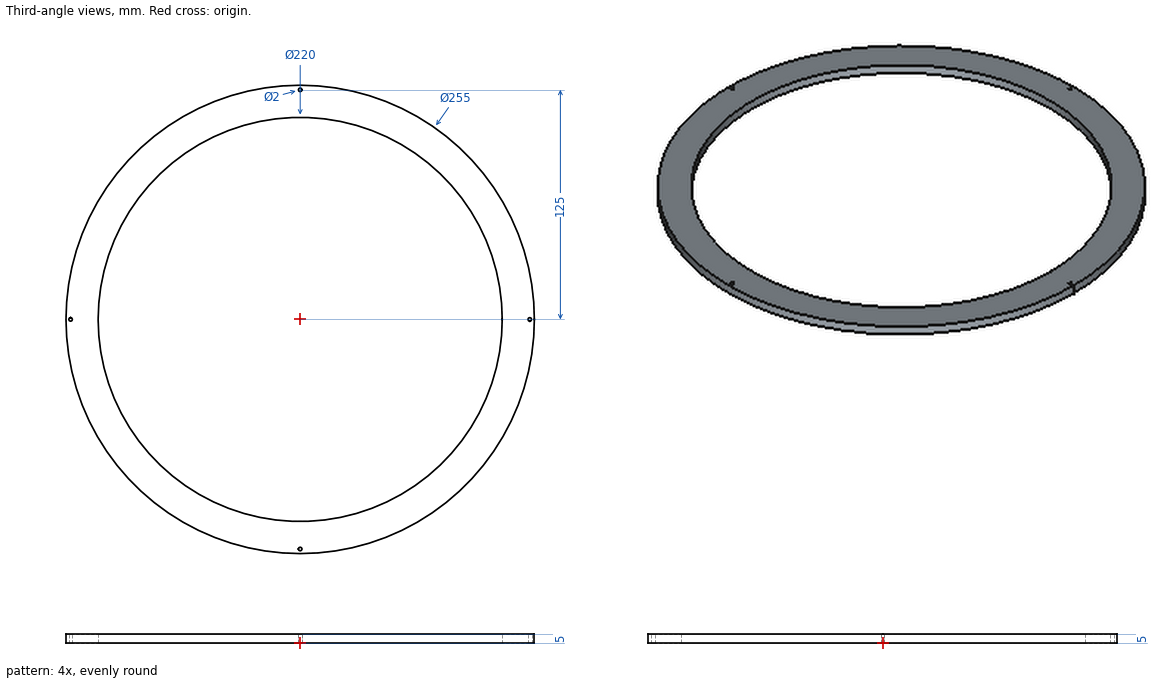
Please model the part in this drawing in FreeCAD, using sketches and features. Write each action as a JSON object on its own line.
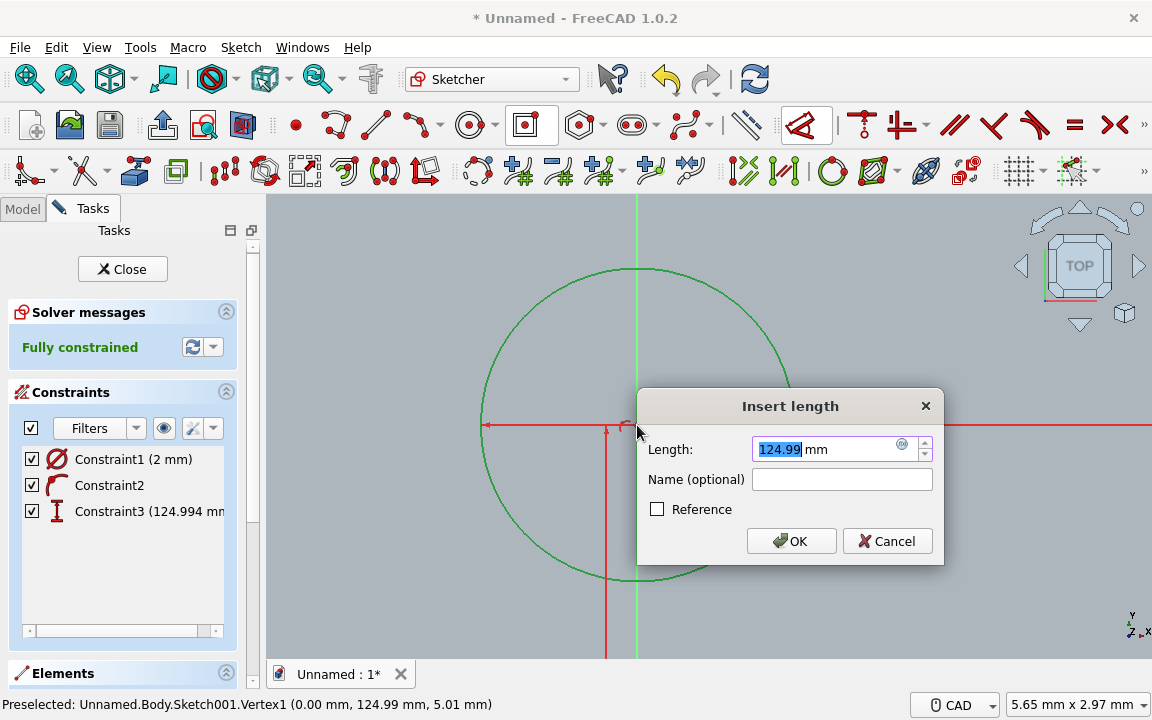
{"action": "type", "text": "125"}
{"action": "key", "text": "Return"}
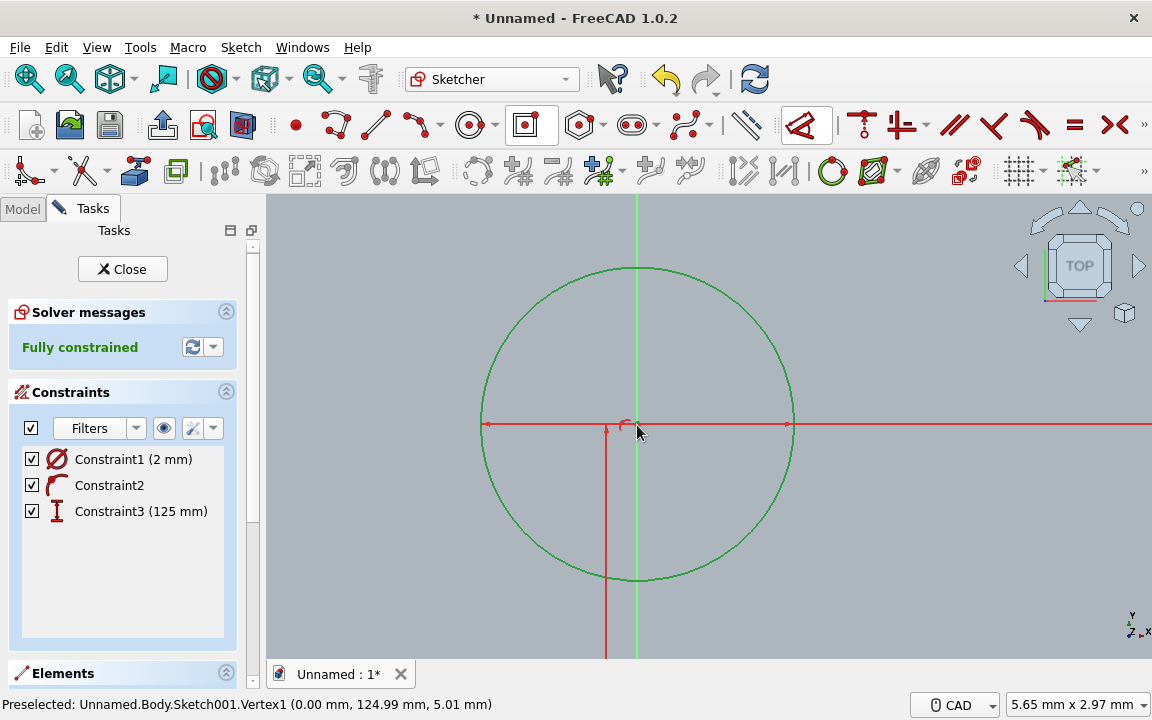
{"action": "left_click", "coordinate": [123, 269]}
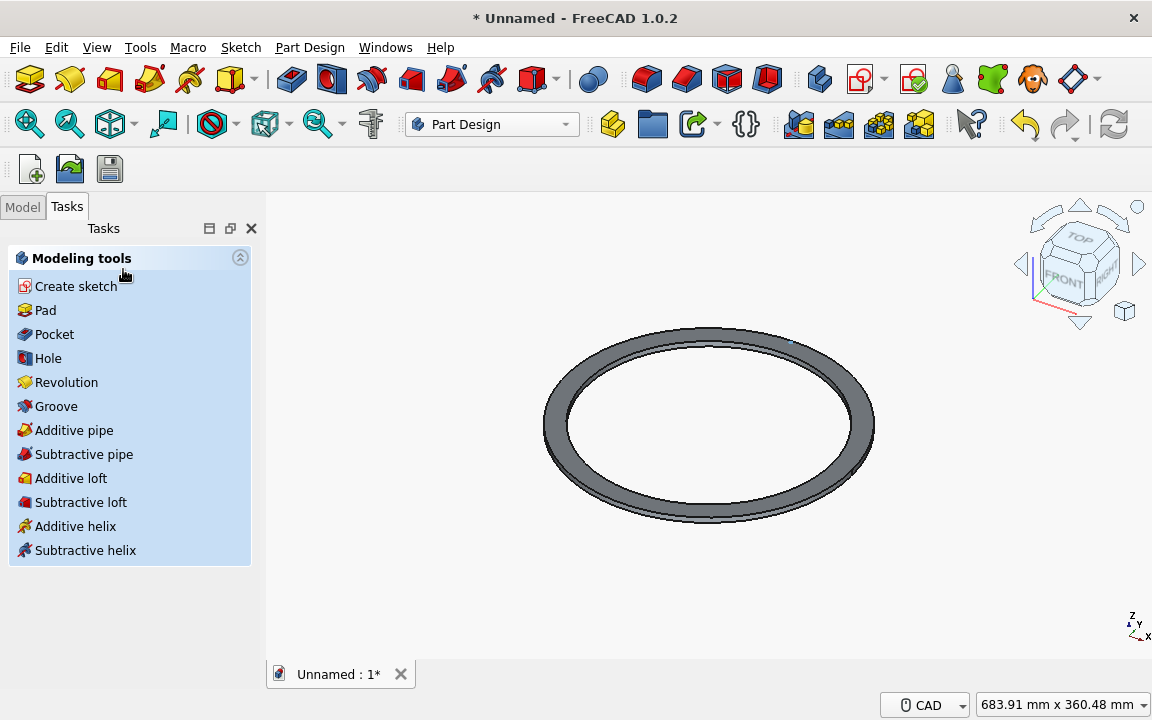
{"action": "left_click", "coordinate": [292, 80]}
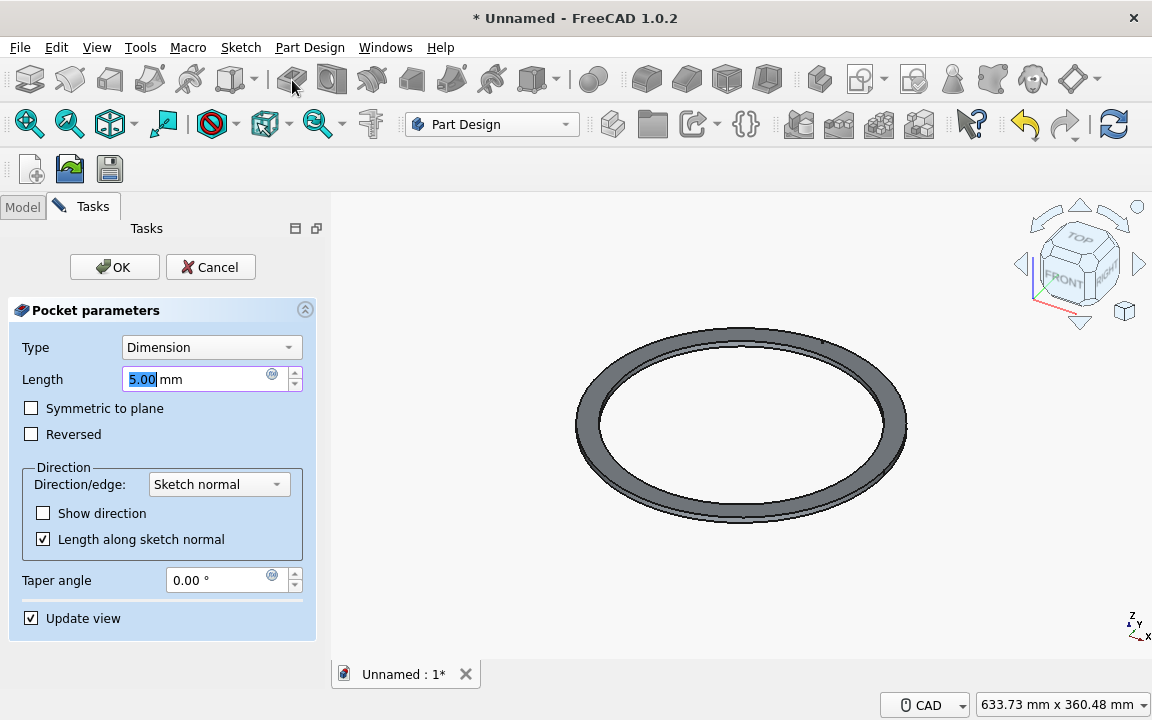
{"action": "type", "text": "5"}
{"action": "key", "text": "Tab"}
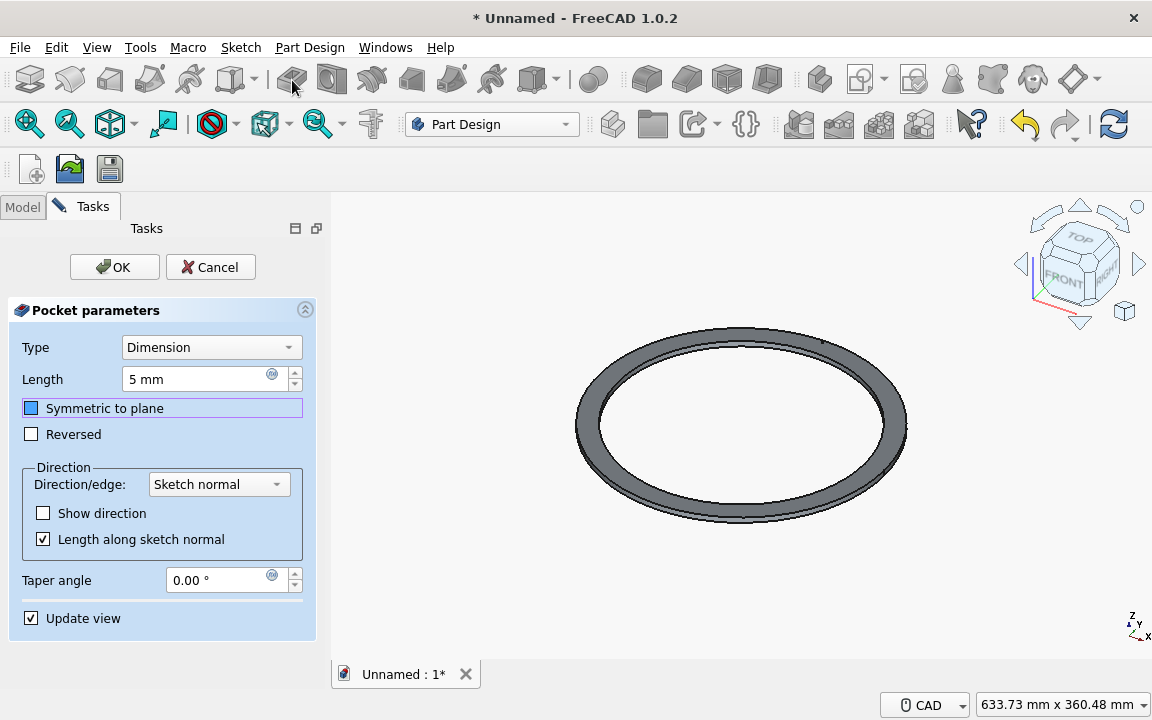
{"action": "left_click", "coordinate": [115, 267]}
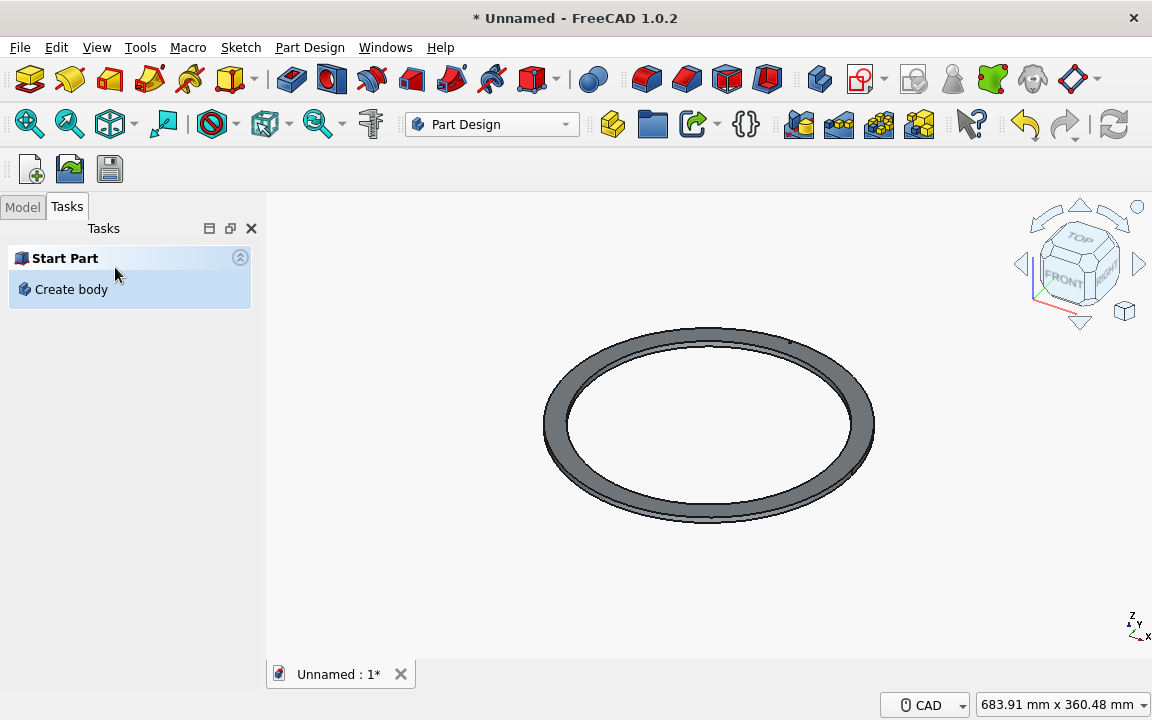
{"action": "left_click", "coordinate": [23, 206]}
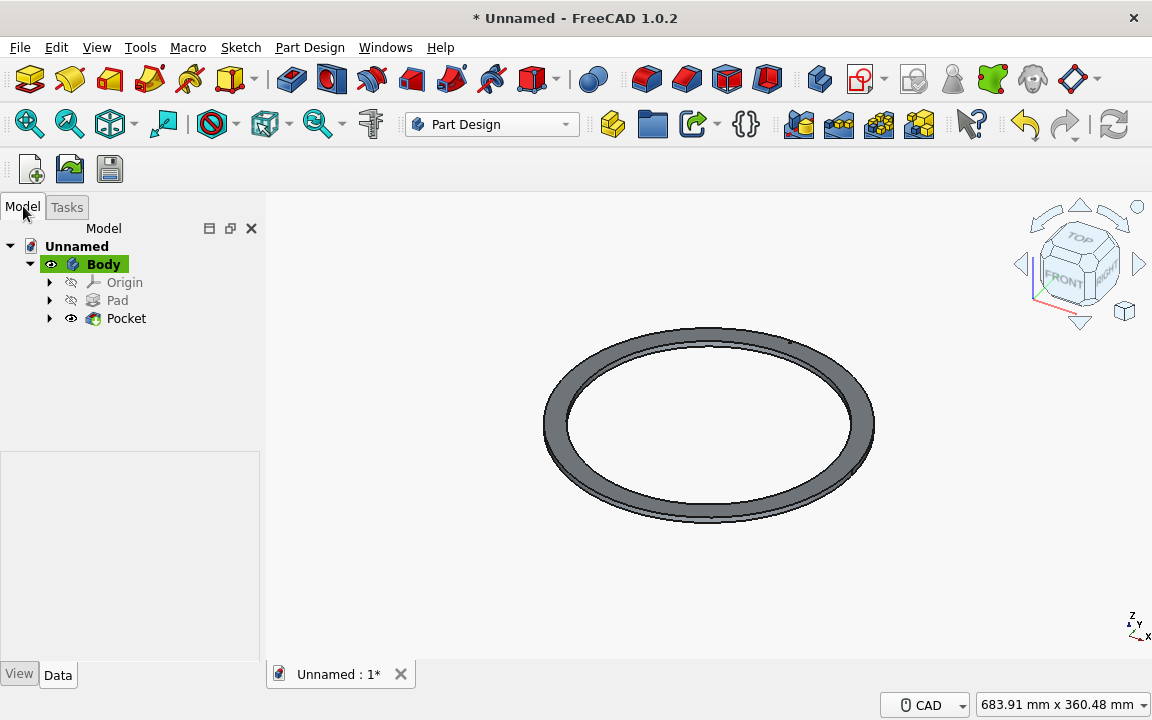
{"action": "left_click", "coordinate": [116, 318]}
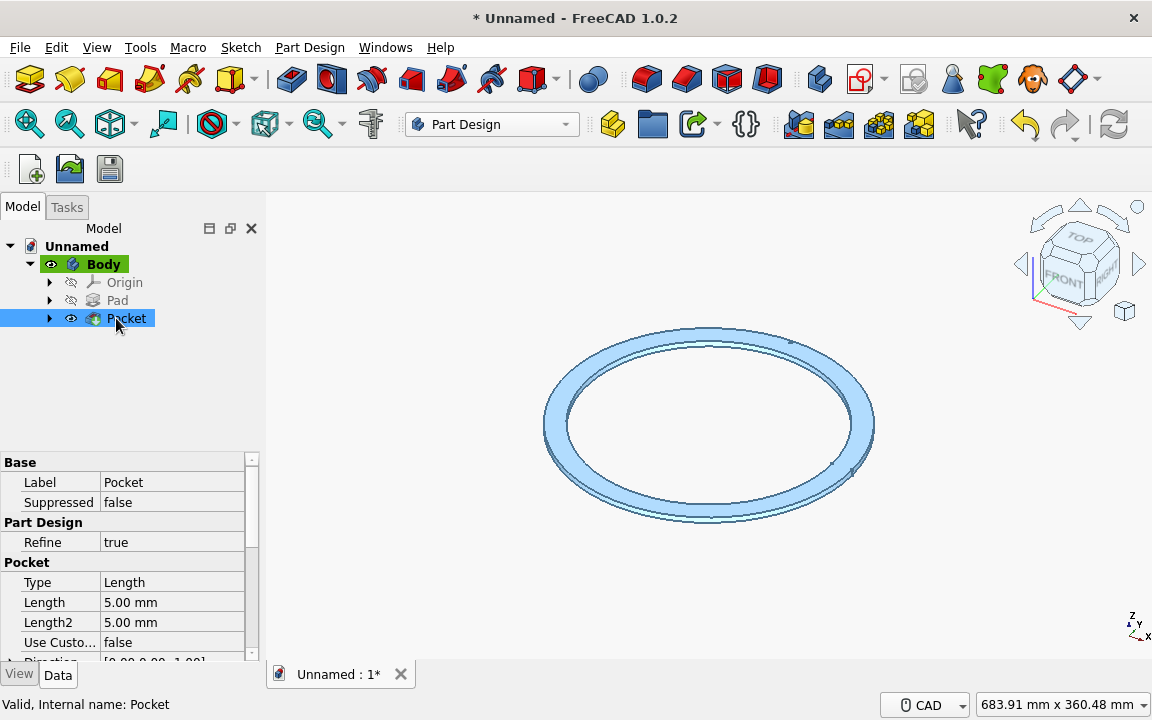
{"action": "left_click", "coordinate": [880, 124]}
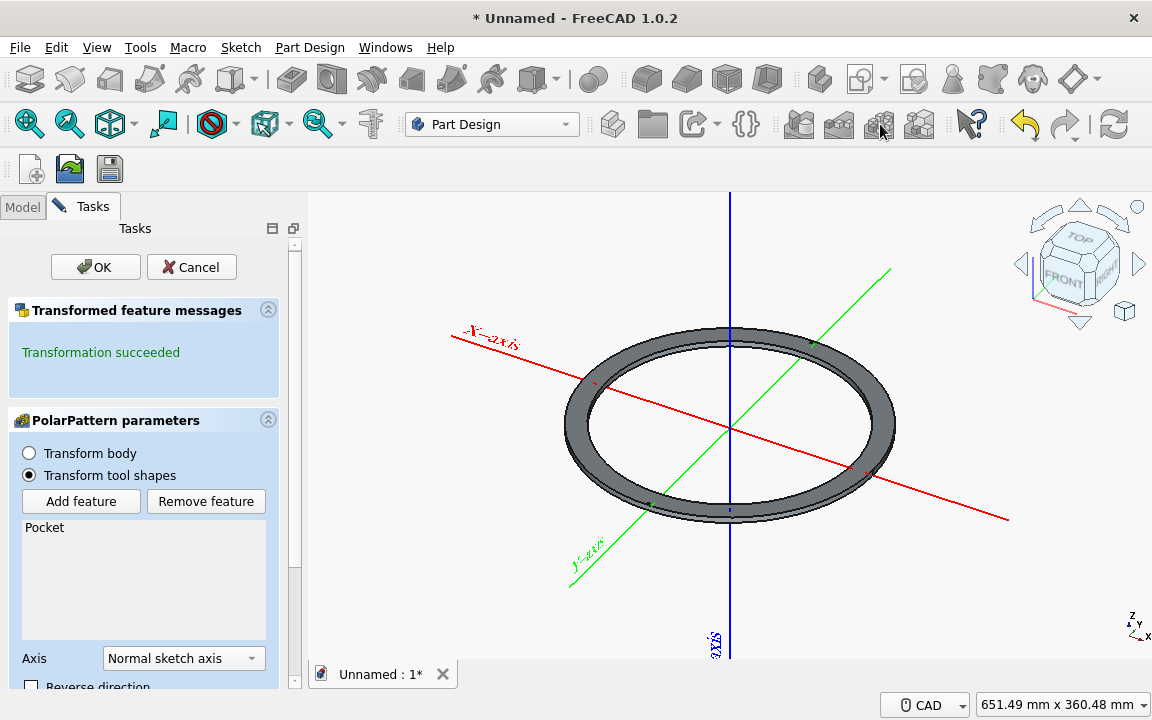
{"action": "left_click", "coordinate": [184, 658]}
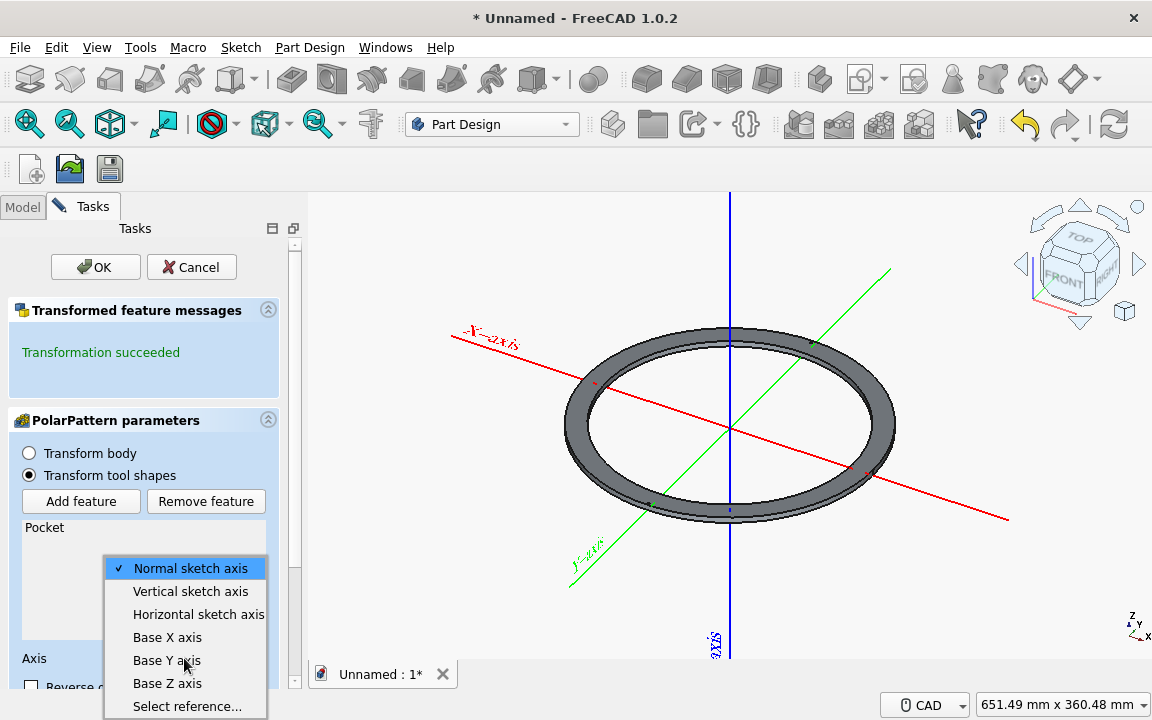
{"action": "left_click", "coordinate": [184, 684]}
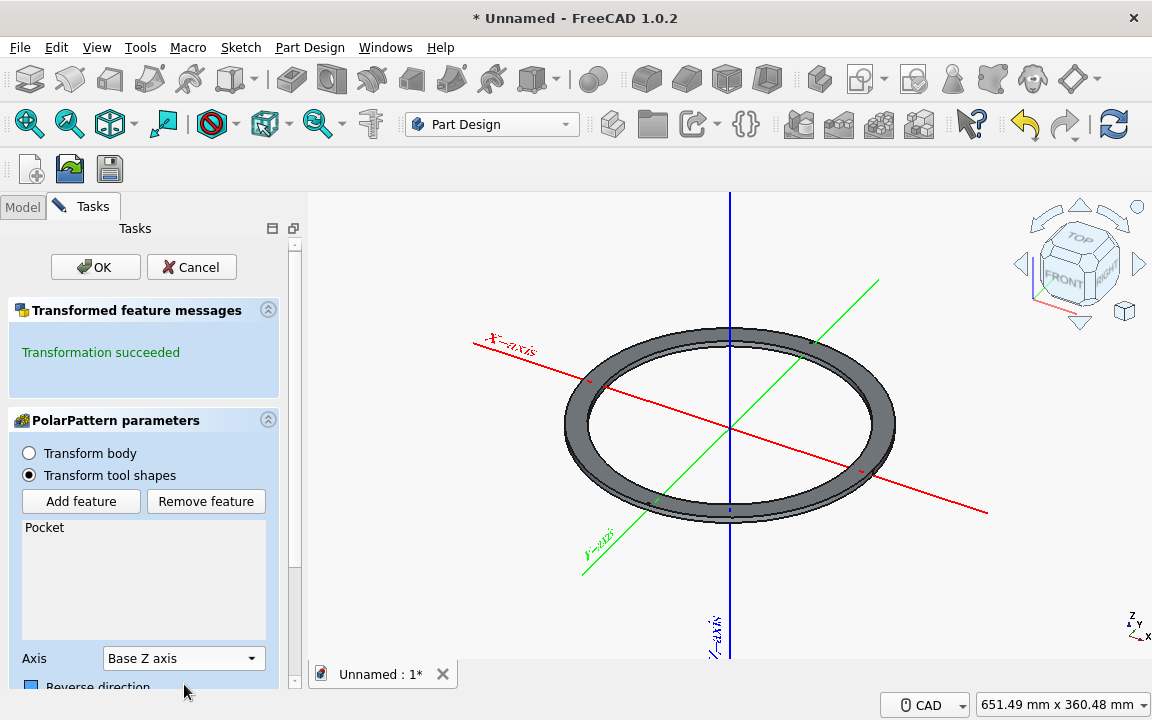
{"action": "scroll", "coordinate": [295, 463], "scroll_direction": "down", "scroll_amount": 3}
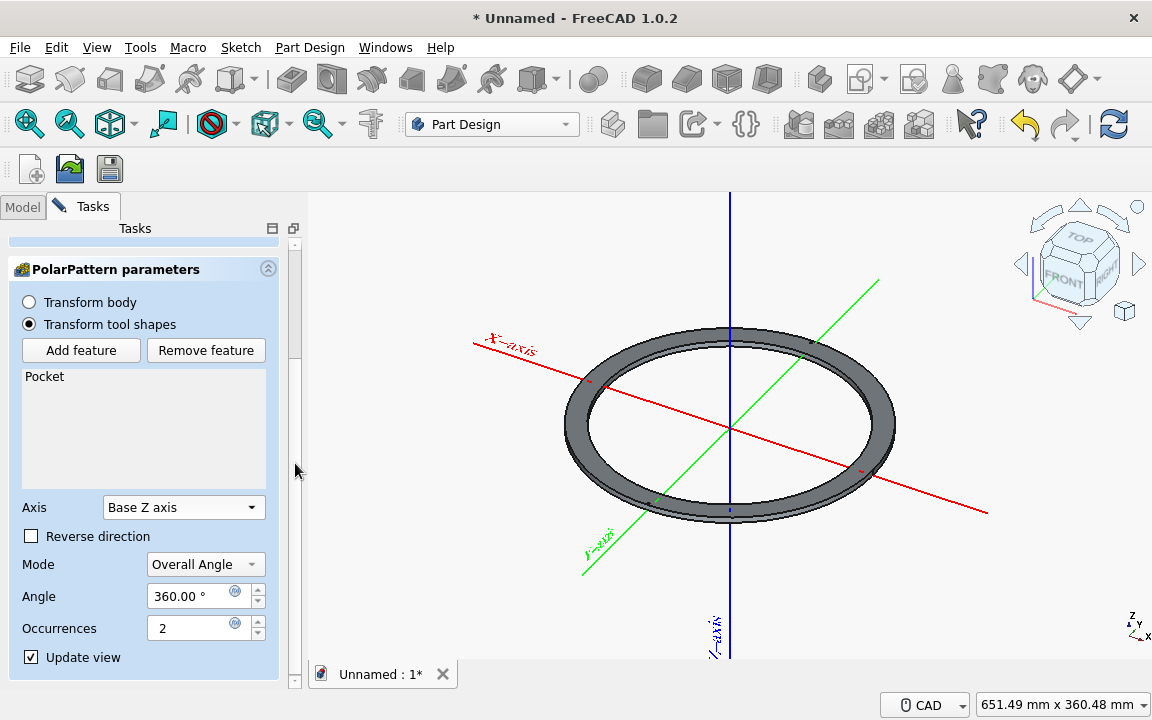
{"action": "triple_click", "coordinate": [198, 628]}